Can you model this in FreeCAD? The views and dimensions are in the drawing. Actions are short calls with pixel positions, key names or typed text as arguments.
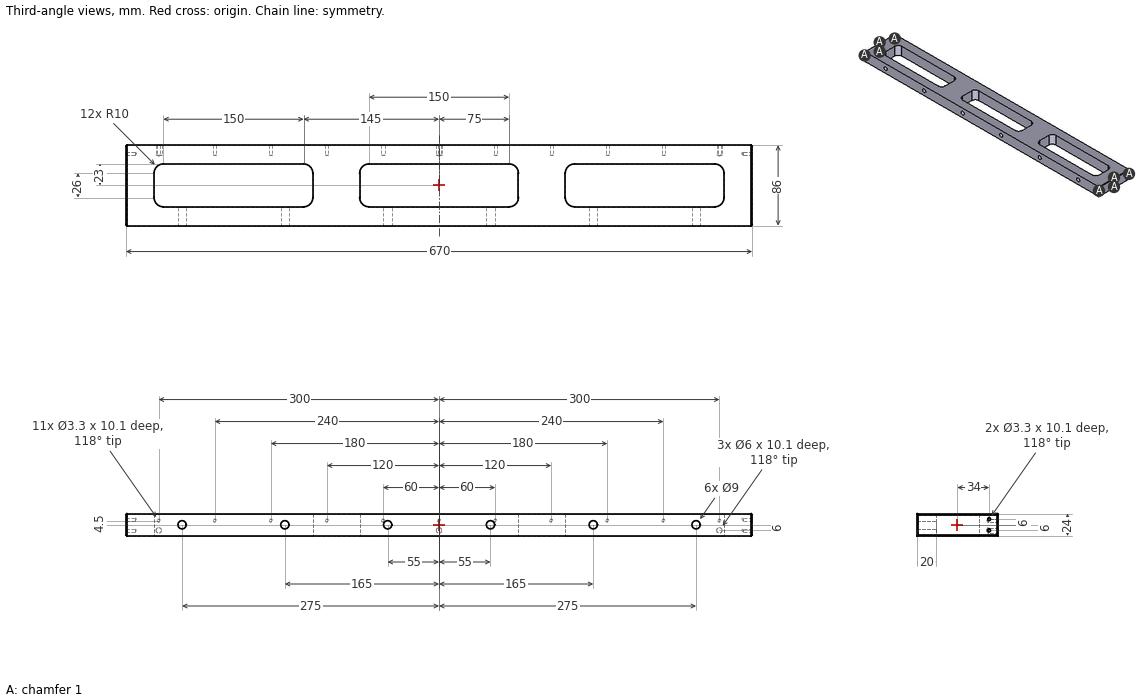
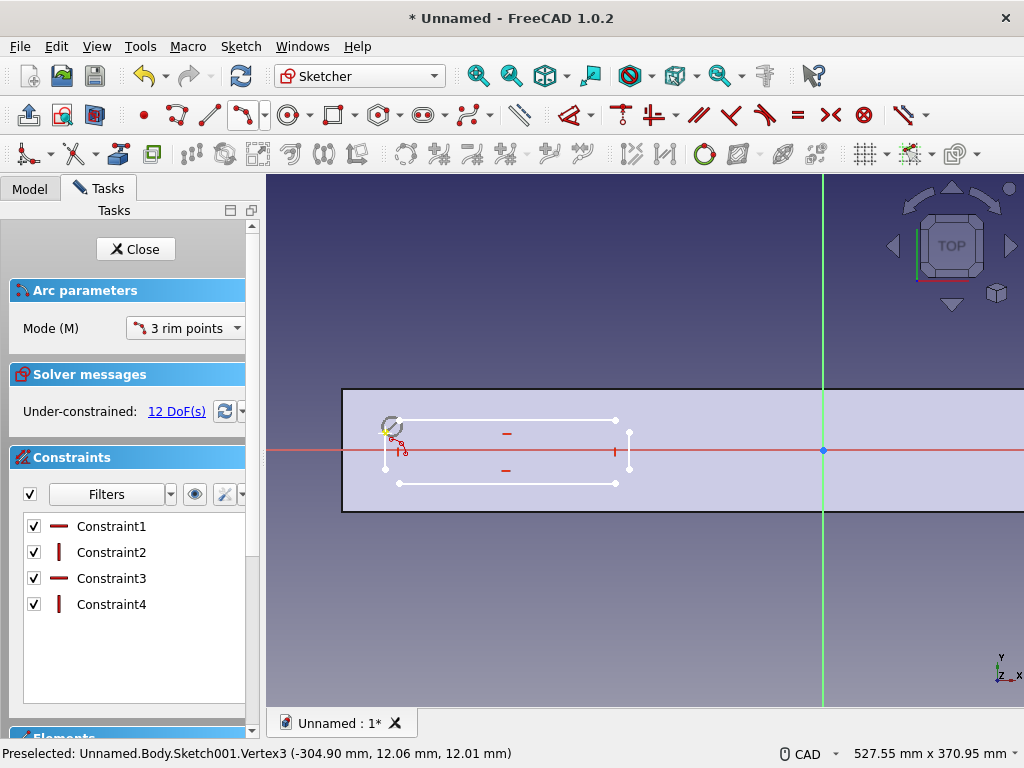
scroll(389, 421, up, 7)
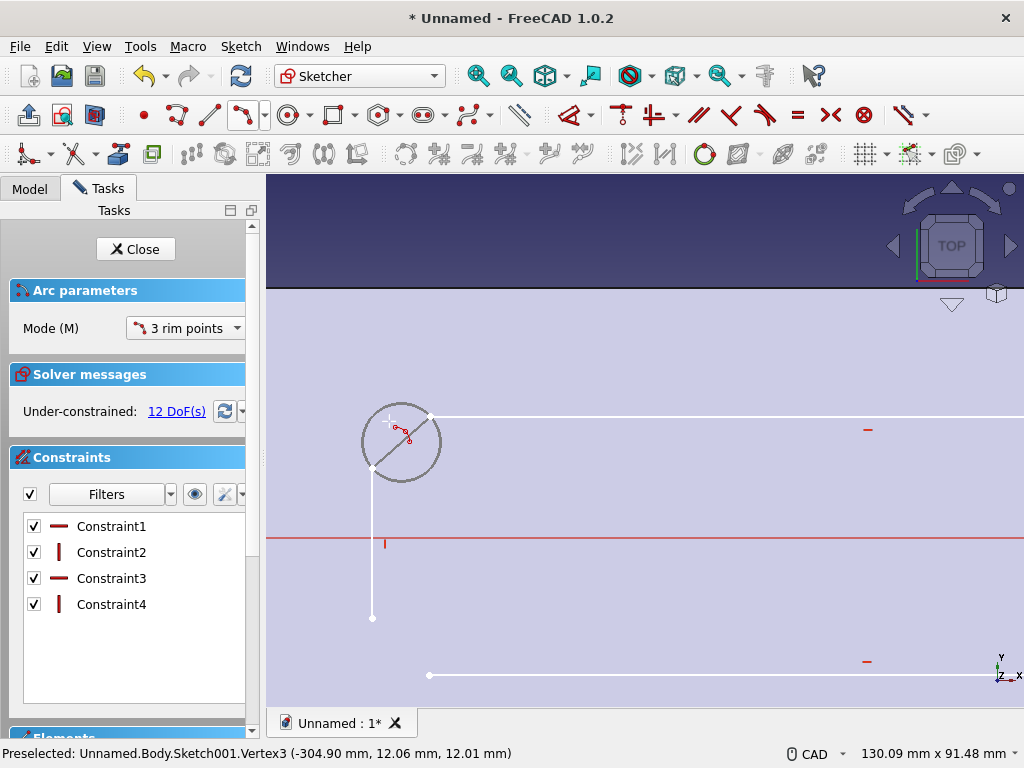
click(389, 422)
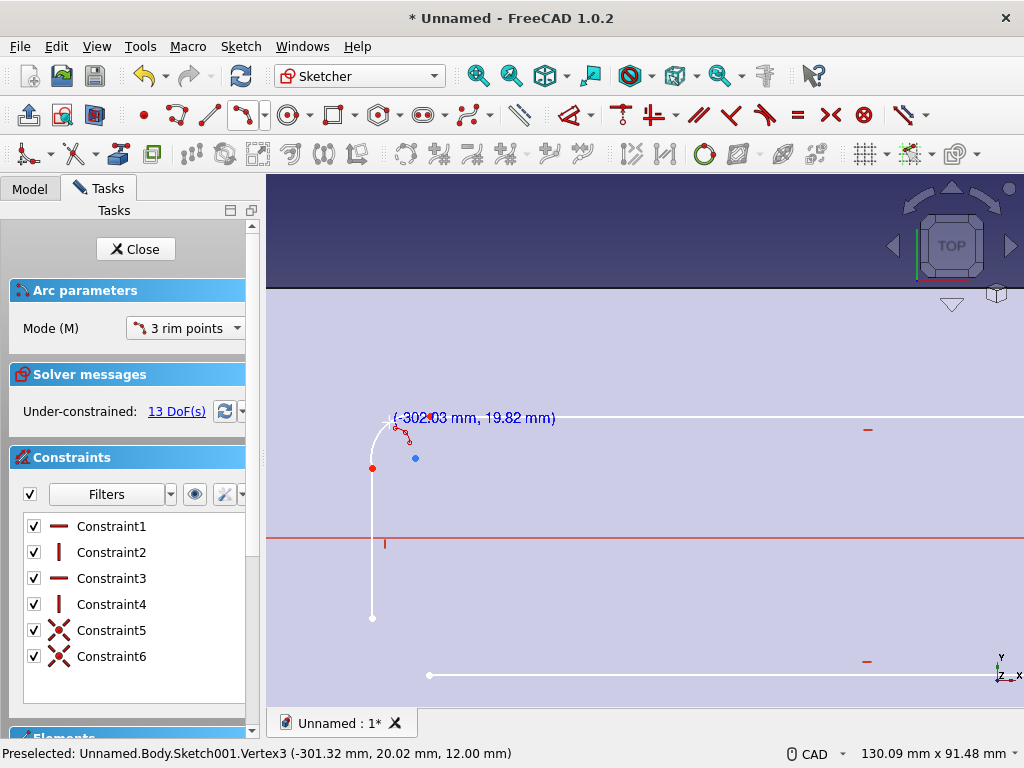
scroll(381, 428, down, 11)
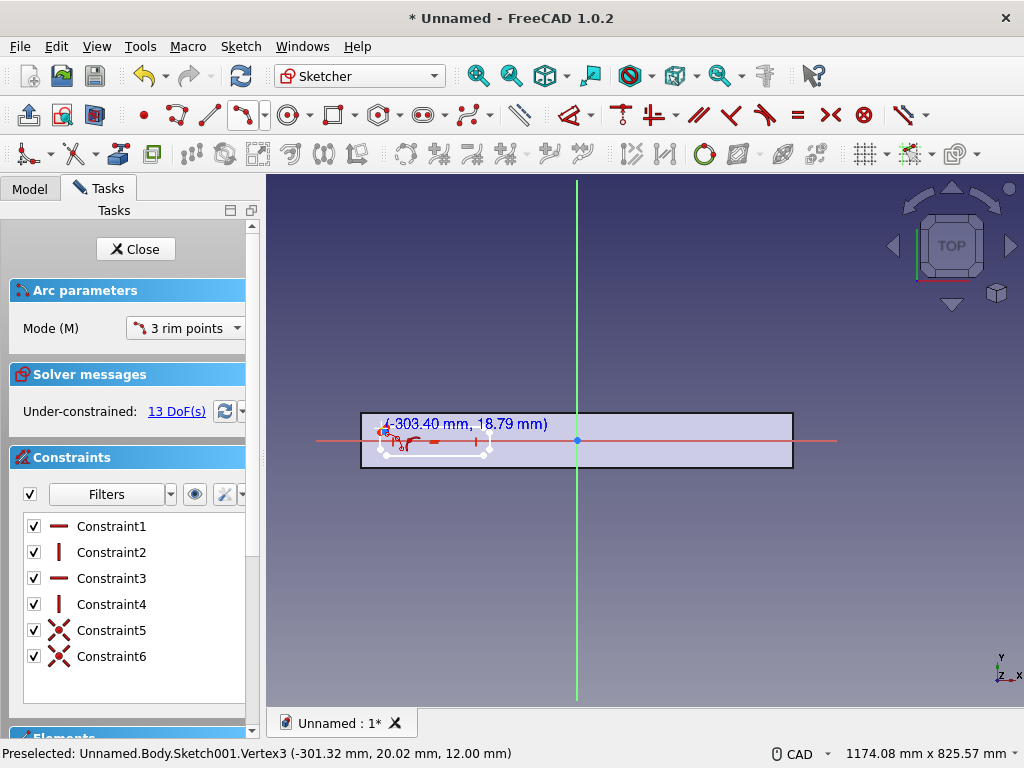
scroll(380, 449, up, 4)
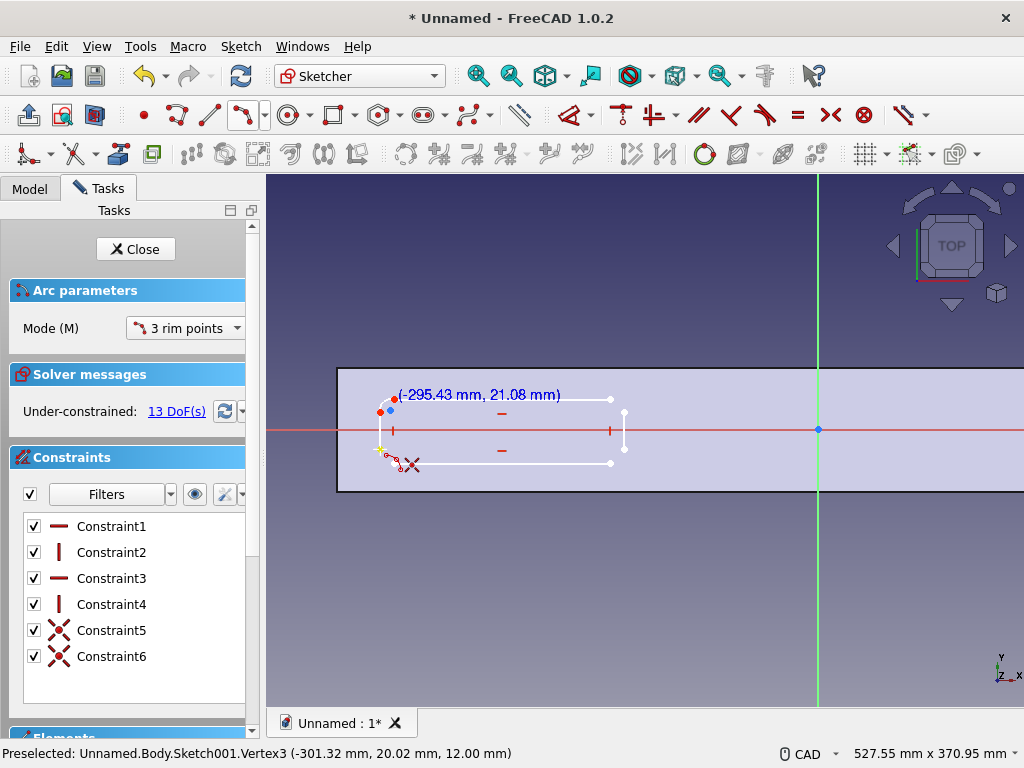
click(380, 449)
click(394, 463)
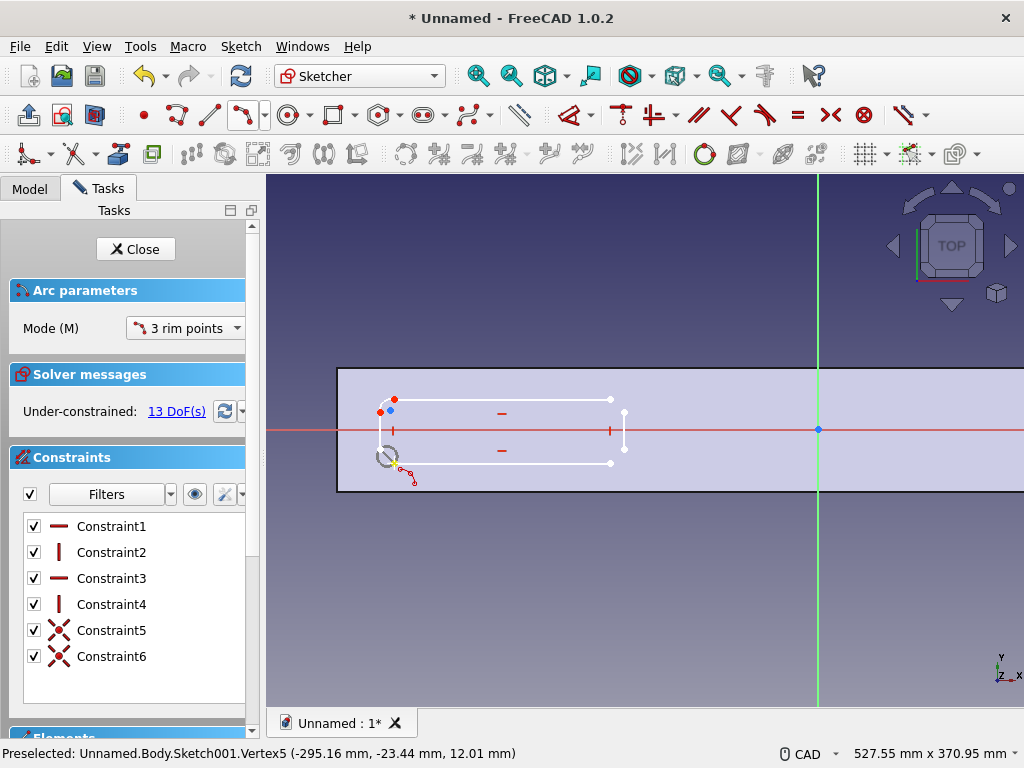
scroll(384, 459, up, 7)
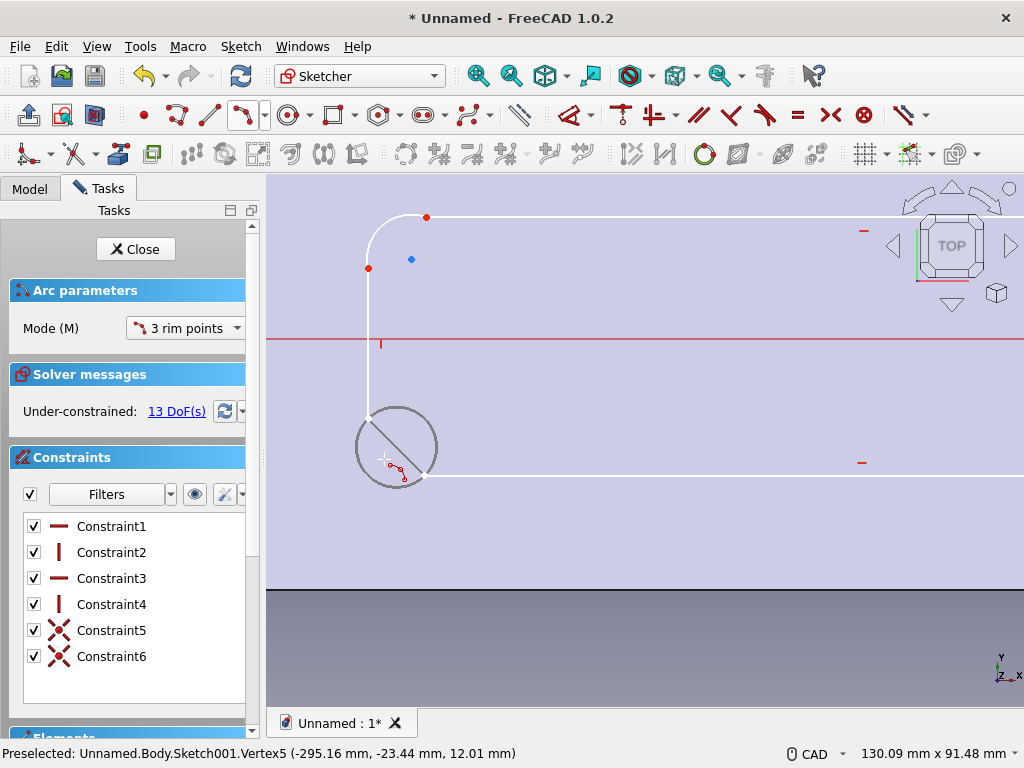
click(385, 456)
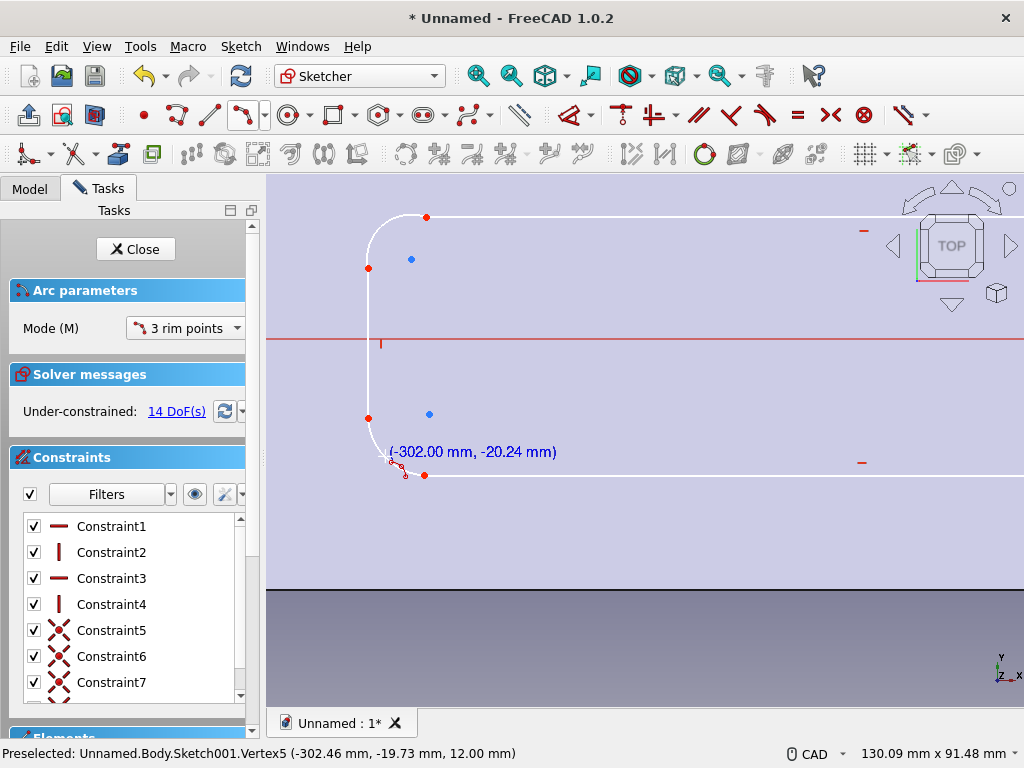
scroll(381, 453, down, 11)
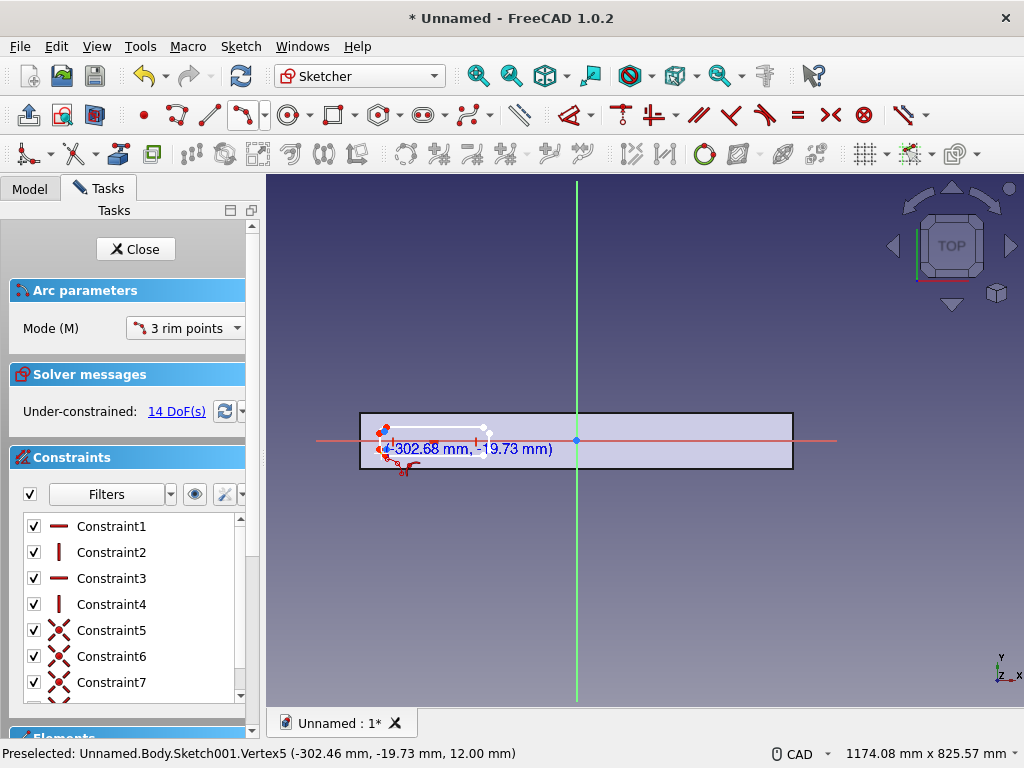
scroll(483, 456, up, 3)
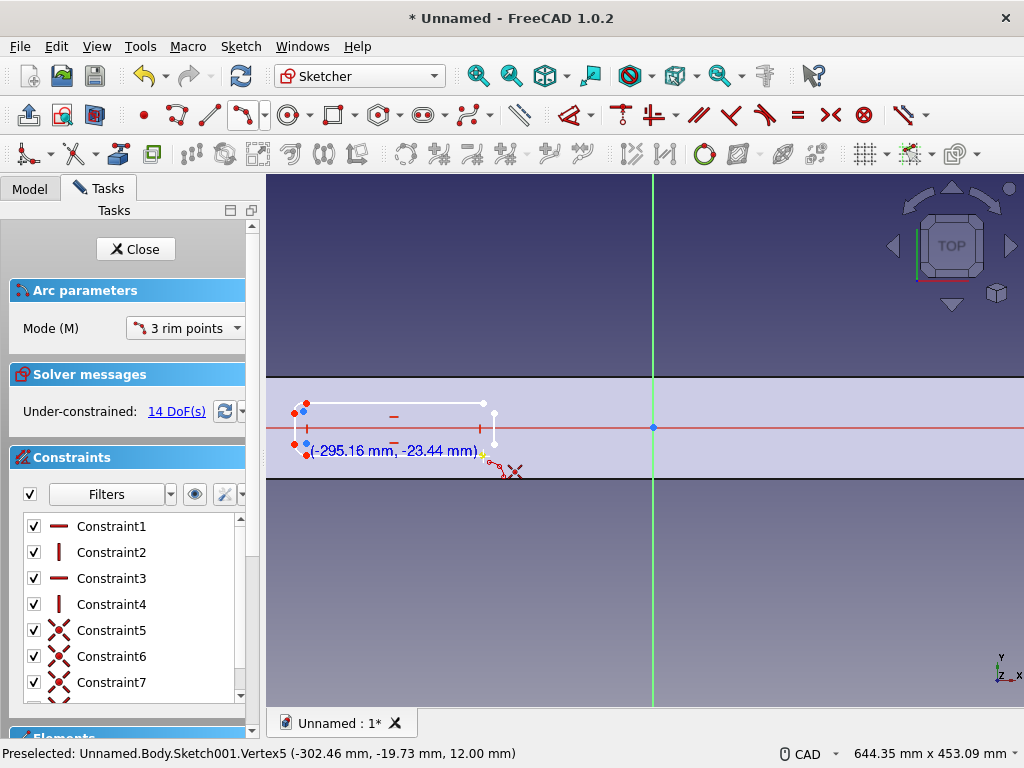
click(483, 456)
click(494, 444)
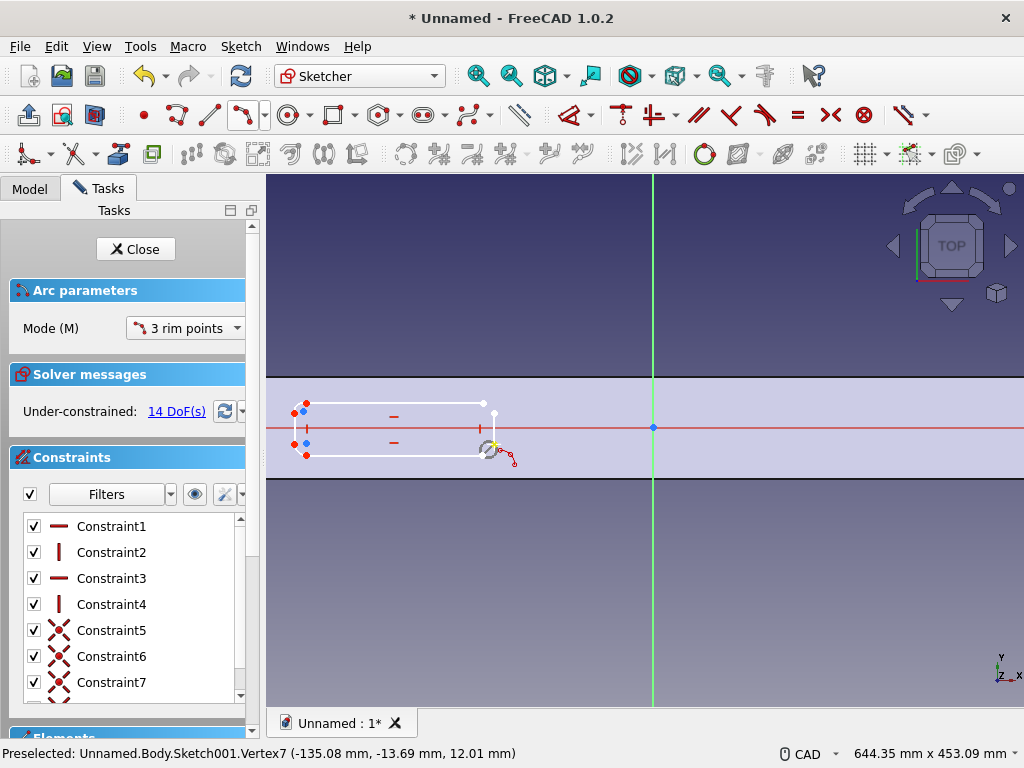
scroll(491, 452, up, 8)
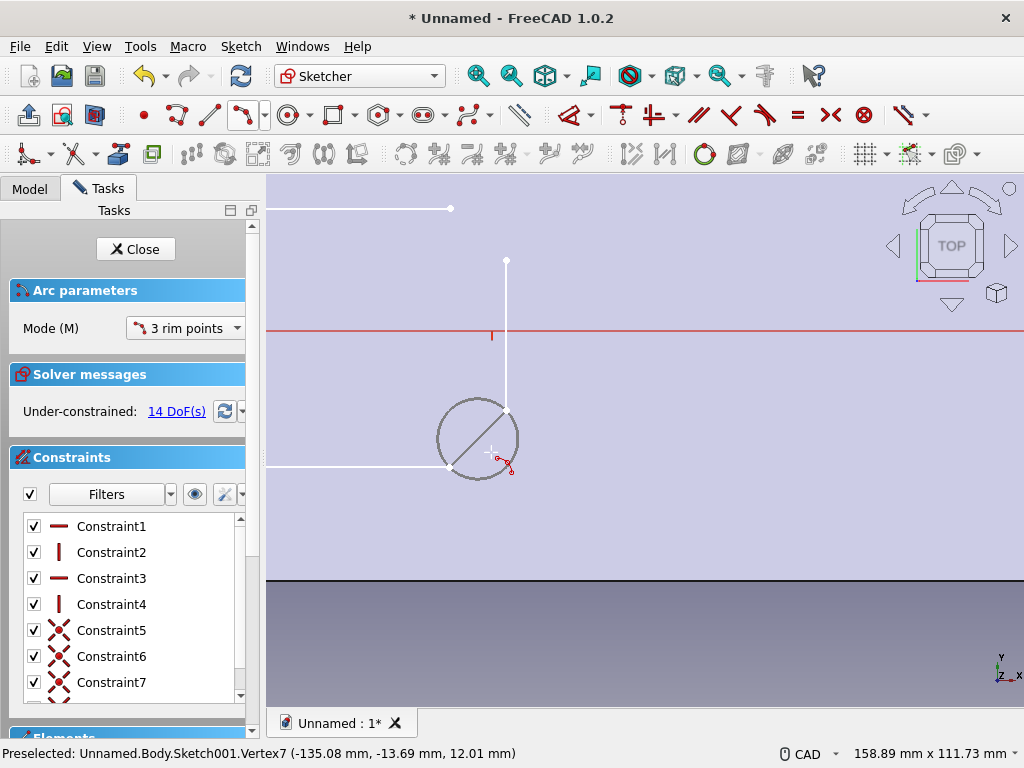
click(490, 448)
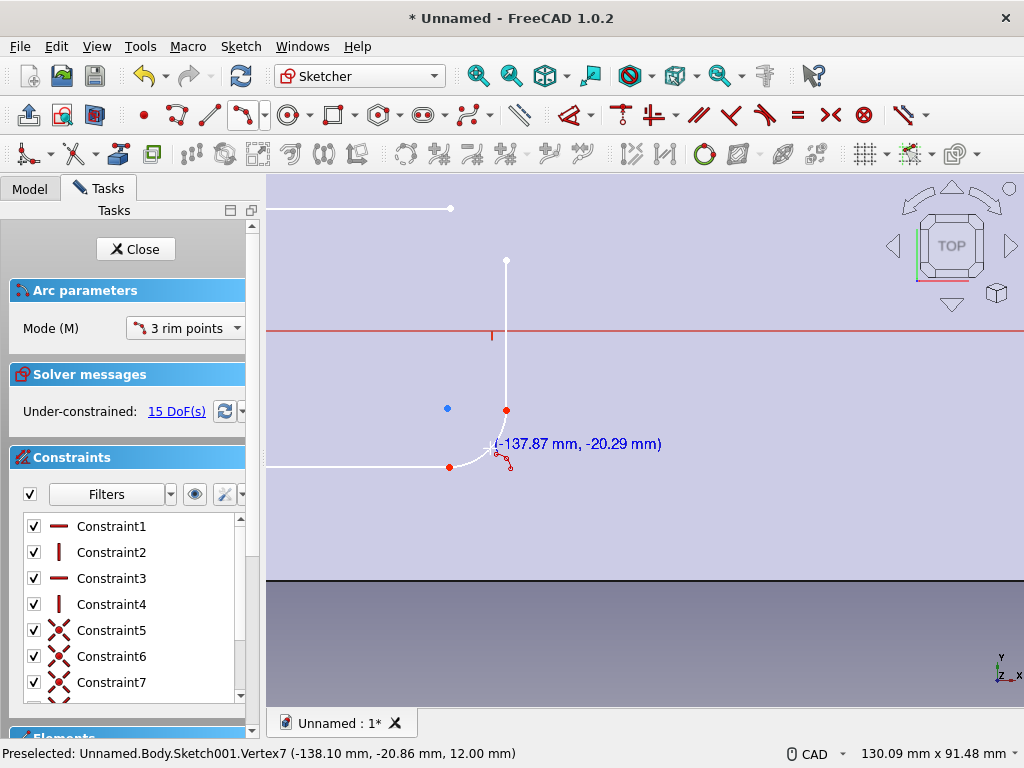
scroll(487, 454, down, 11)